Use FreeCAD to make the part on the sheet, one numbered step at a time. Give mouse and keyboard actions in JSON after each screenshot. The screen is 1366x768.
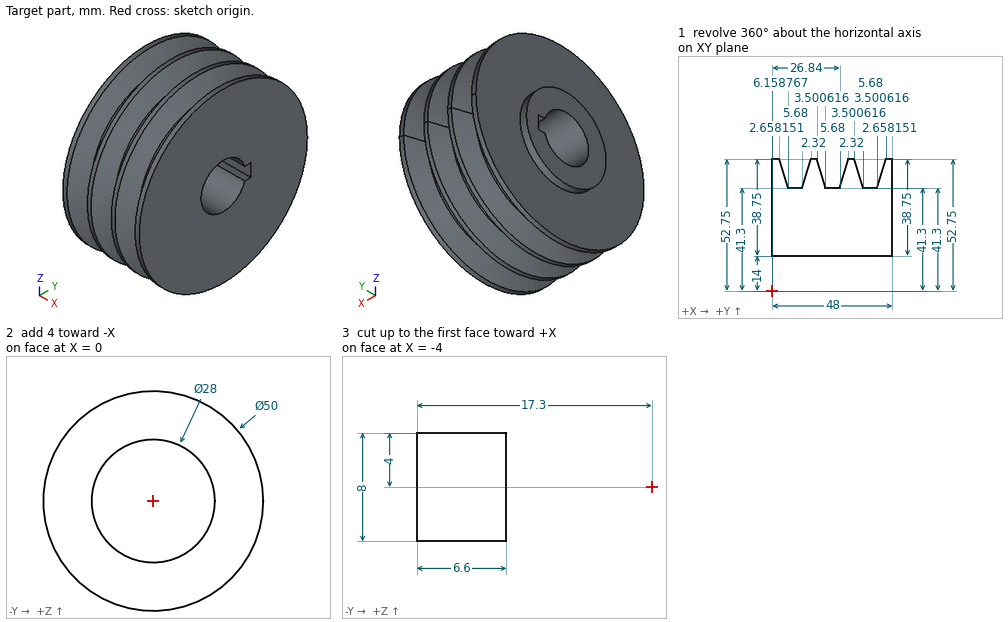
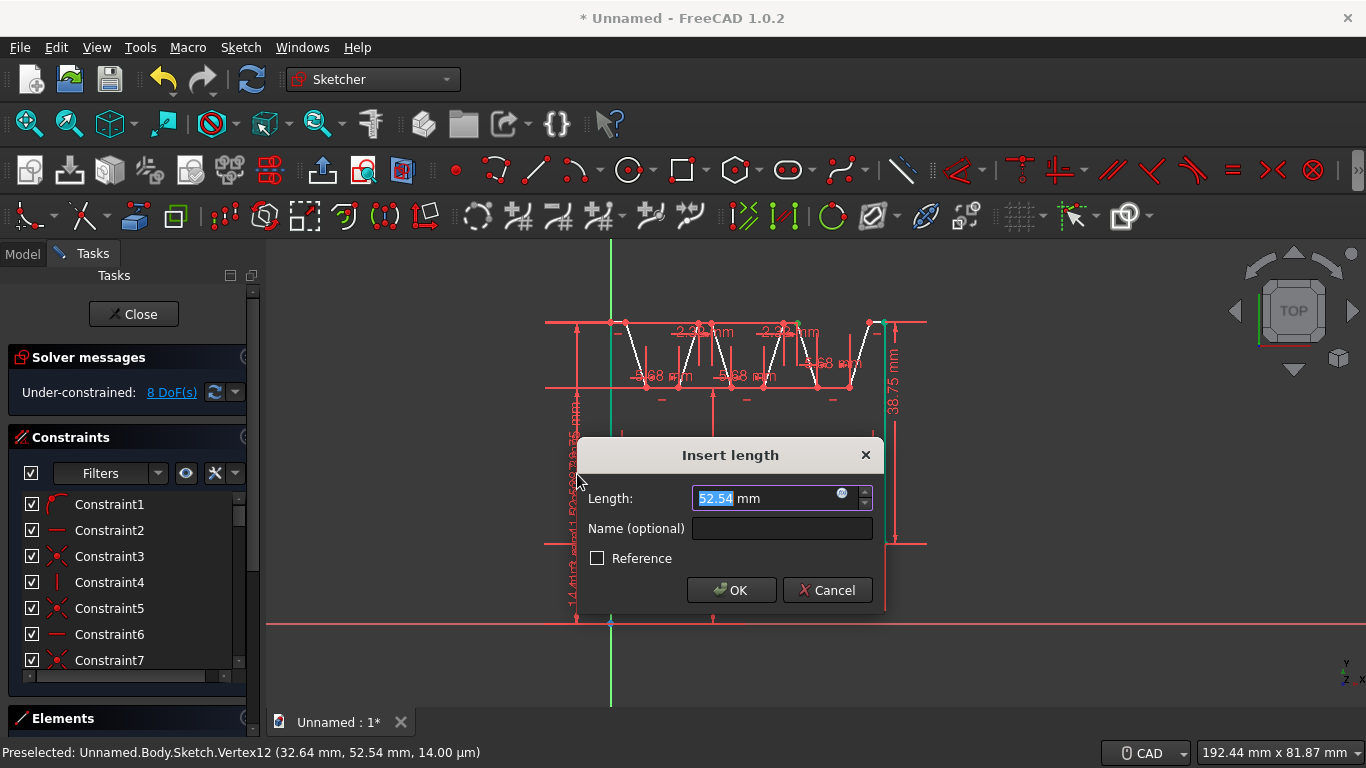
{"action": "type", "text": "52.75"}
{"action": "key", "text": "Return"}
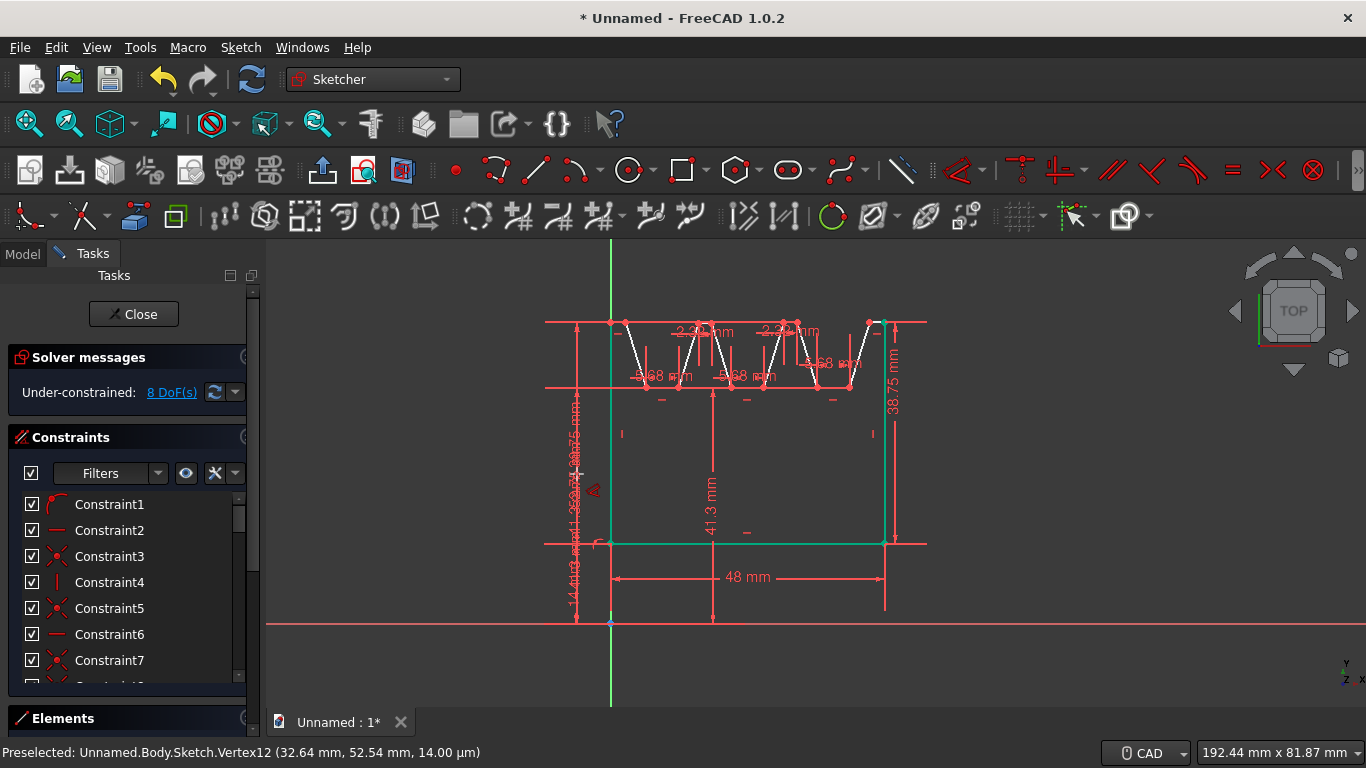
{"action": "left_click", "coordinate": [764, 388]}
{"action": "left_click", "coordinate": [687, 658]}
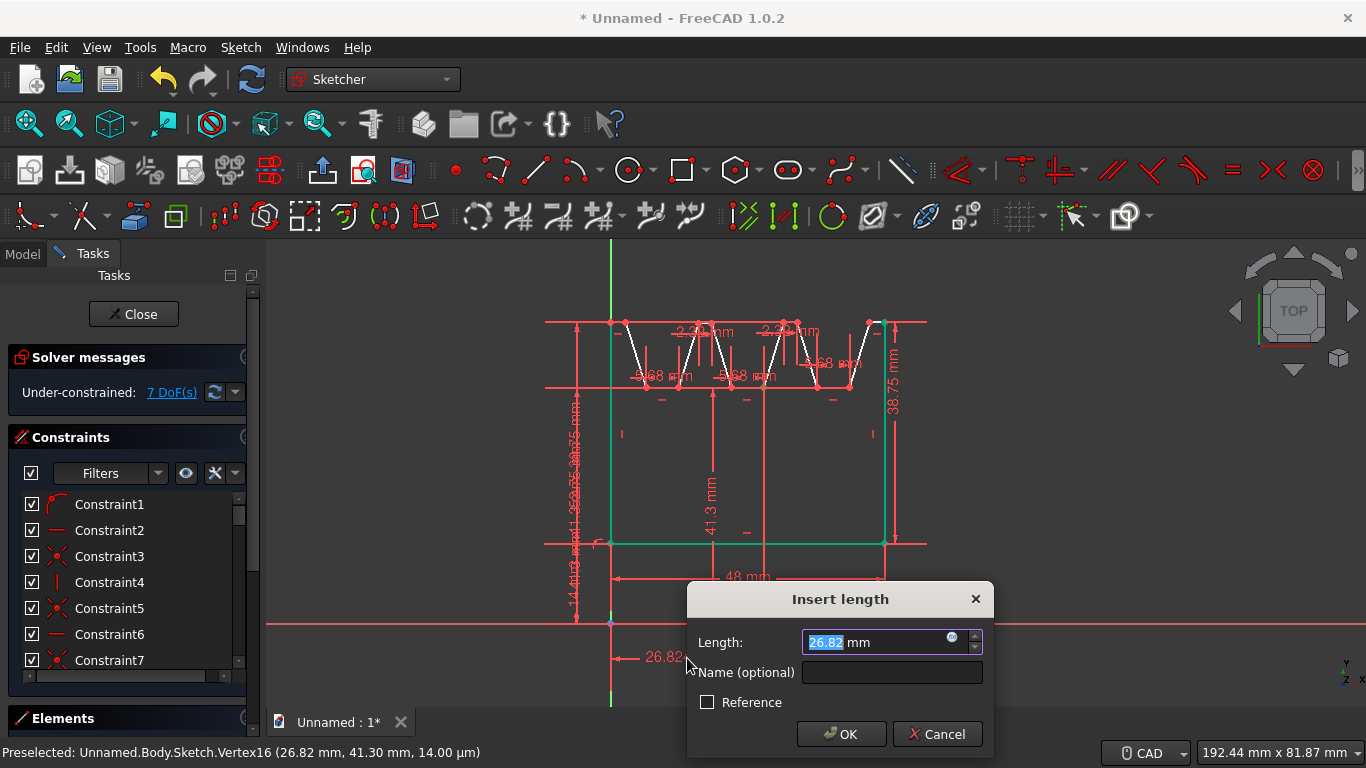
{"action": "type", "text": "26.84"}
{"action": "key", "text": "Return"}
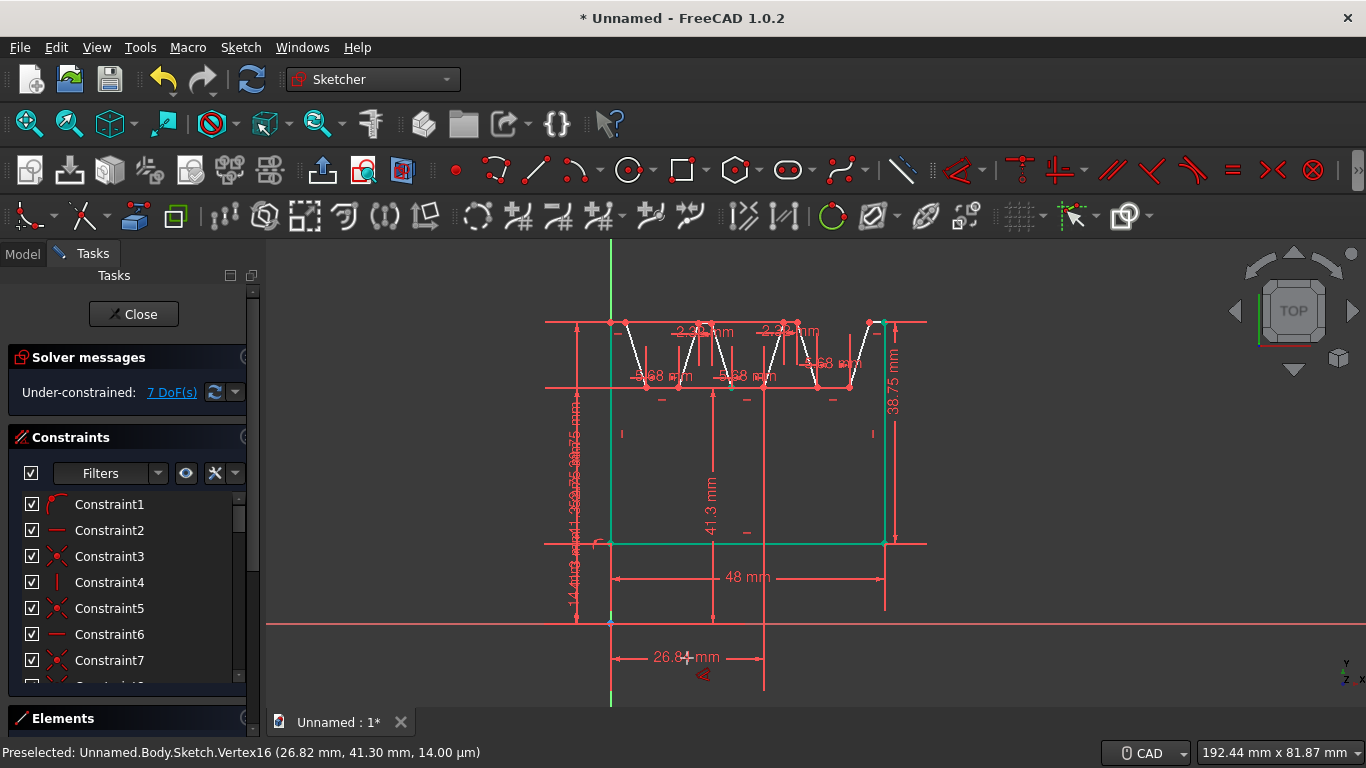
{"action": "left_click", "coordinate": [712, 323]}
{"action": "left_click", "coordinate": [577, 405]}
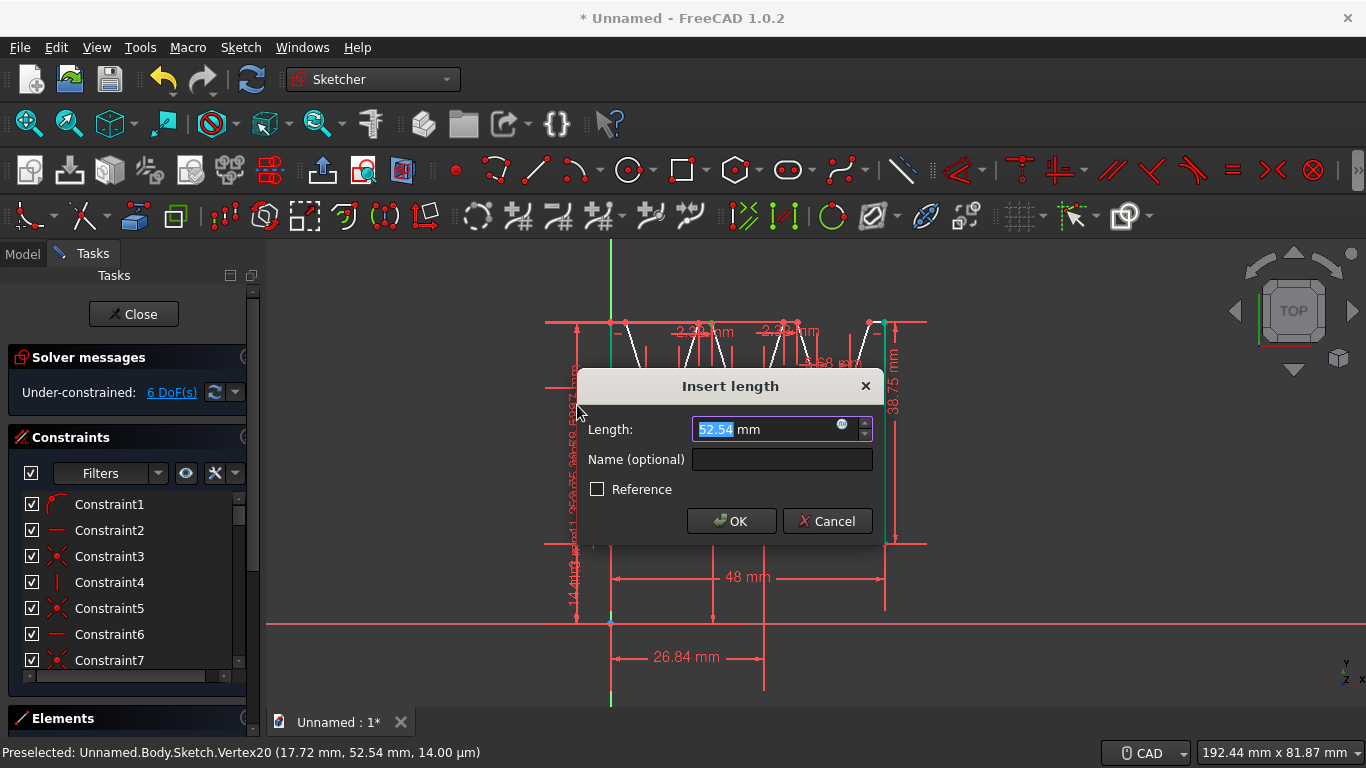
{"action": "type", "text": "52.75"}
{"action": "key", "text": "Return"}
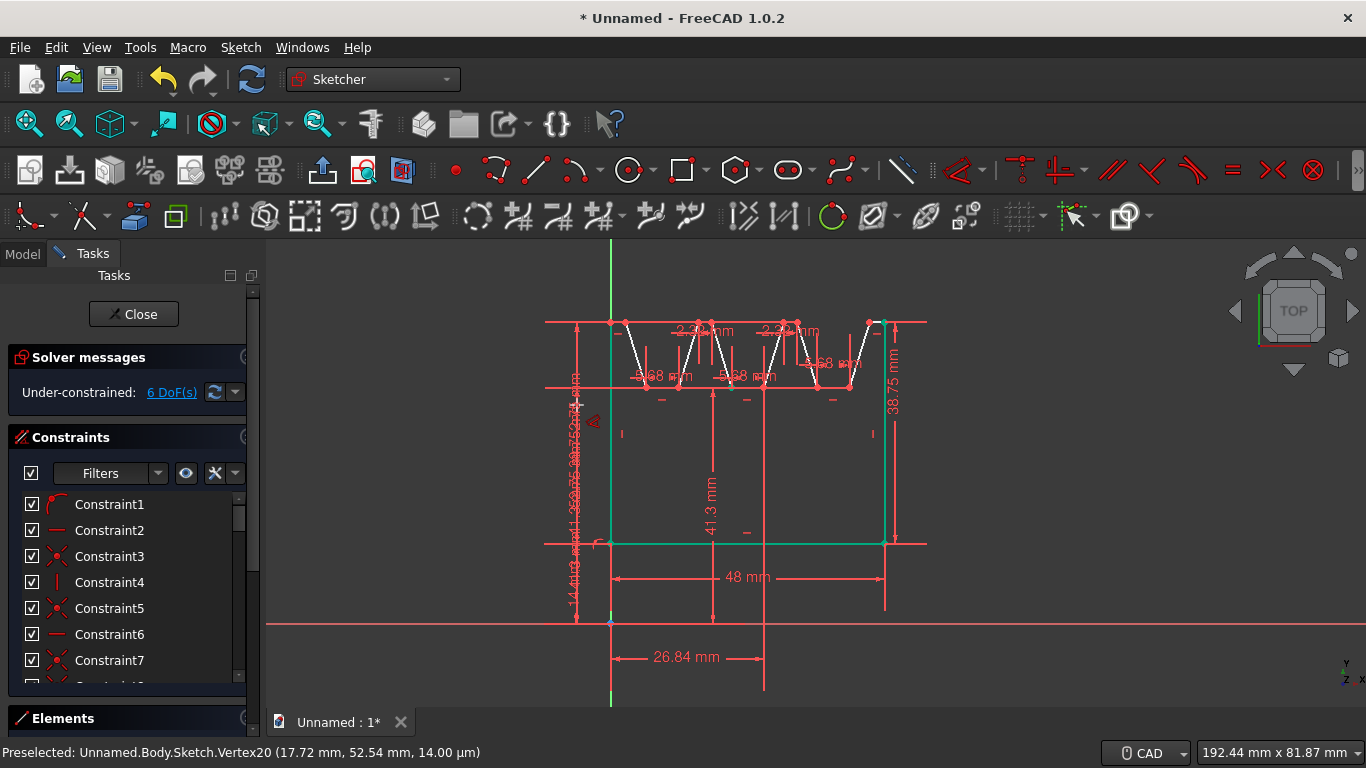
{"action": "scroll", "coordinate": [877, 322], "scroll_direction": "up", "scroll_amount": 5}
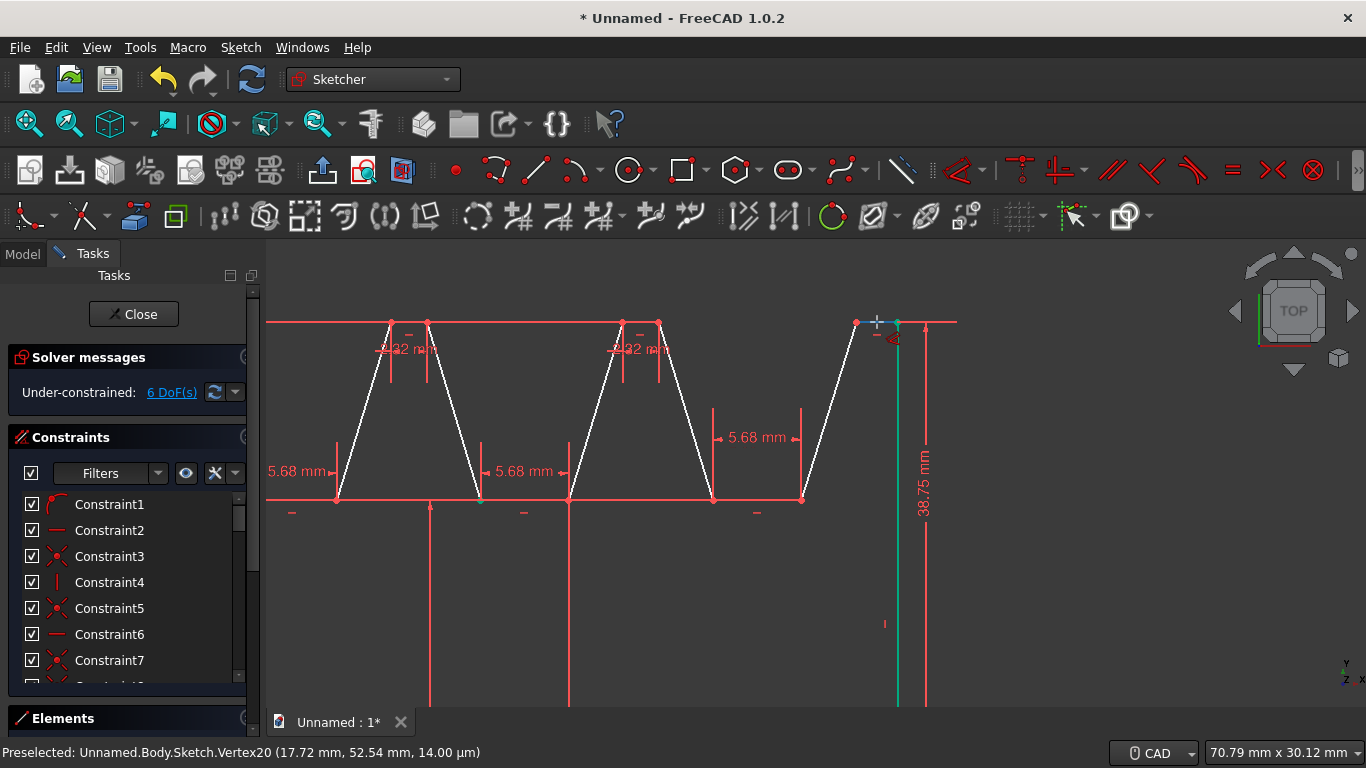
{"action": "left_click", "coordinate": [877, 322]}
{"action": "left_click", "coordinate": [877, 288]}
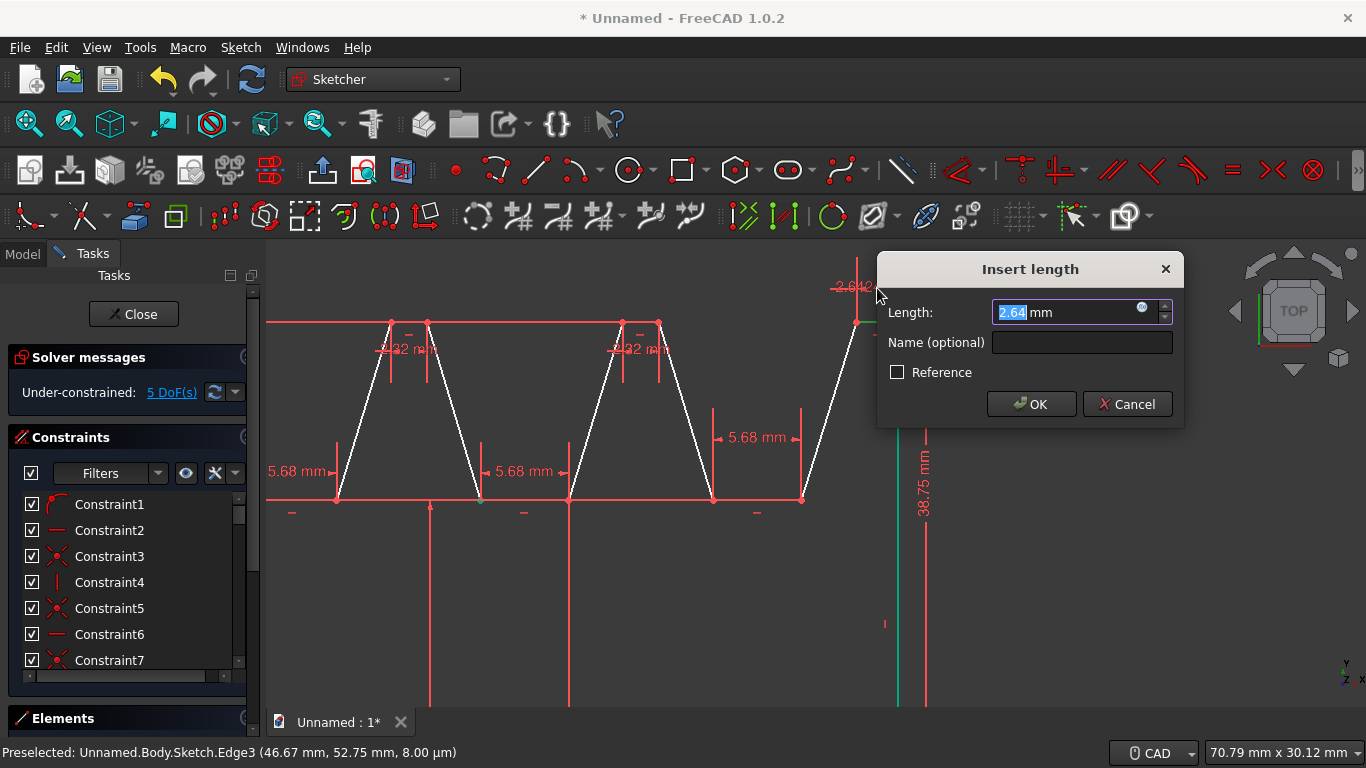
{"action": "type", "text": "2.658151"}
{"action": "key", "text": "Return"}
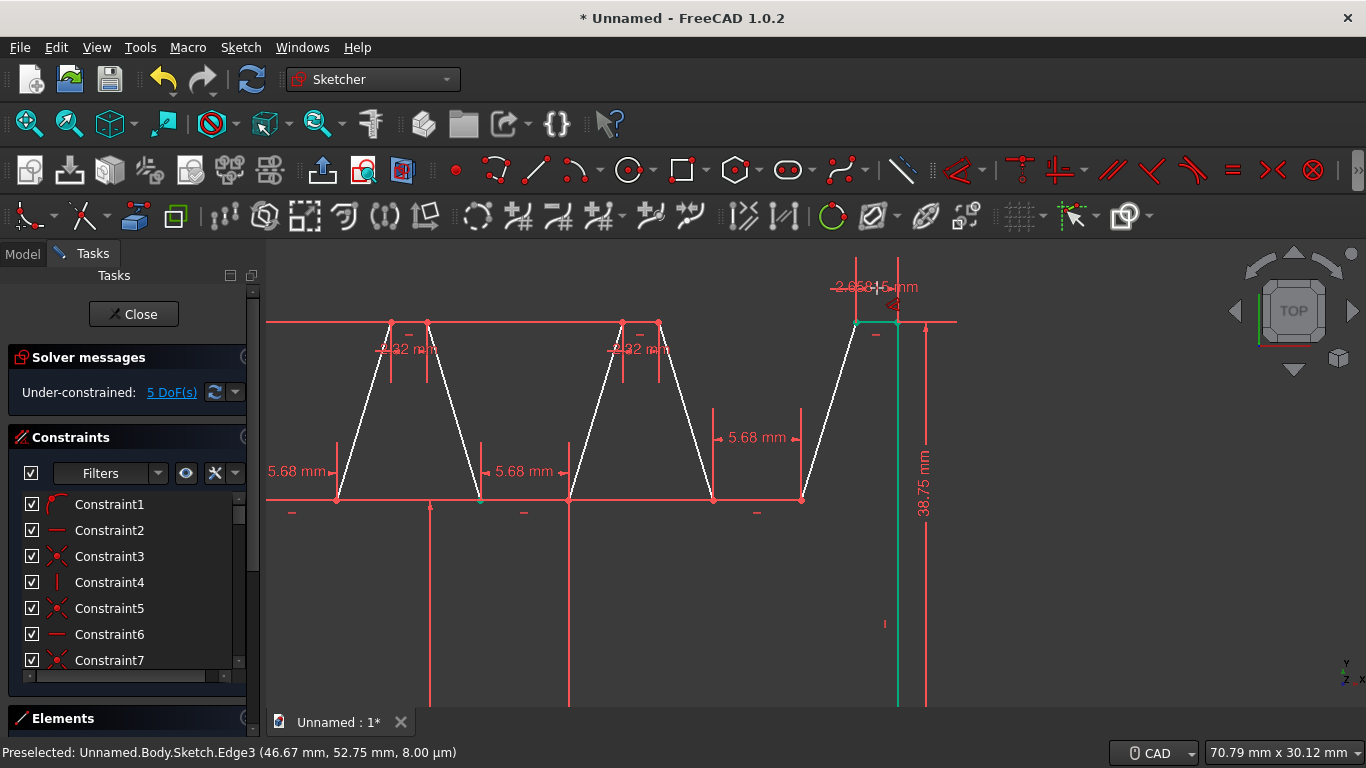
{"action": "scroll", "coordinate": [877, 322], "scroll_direction": "down", "scroll_amount": 5}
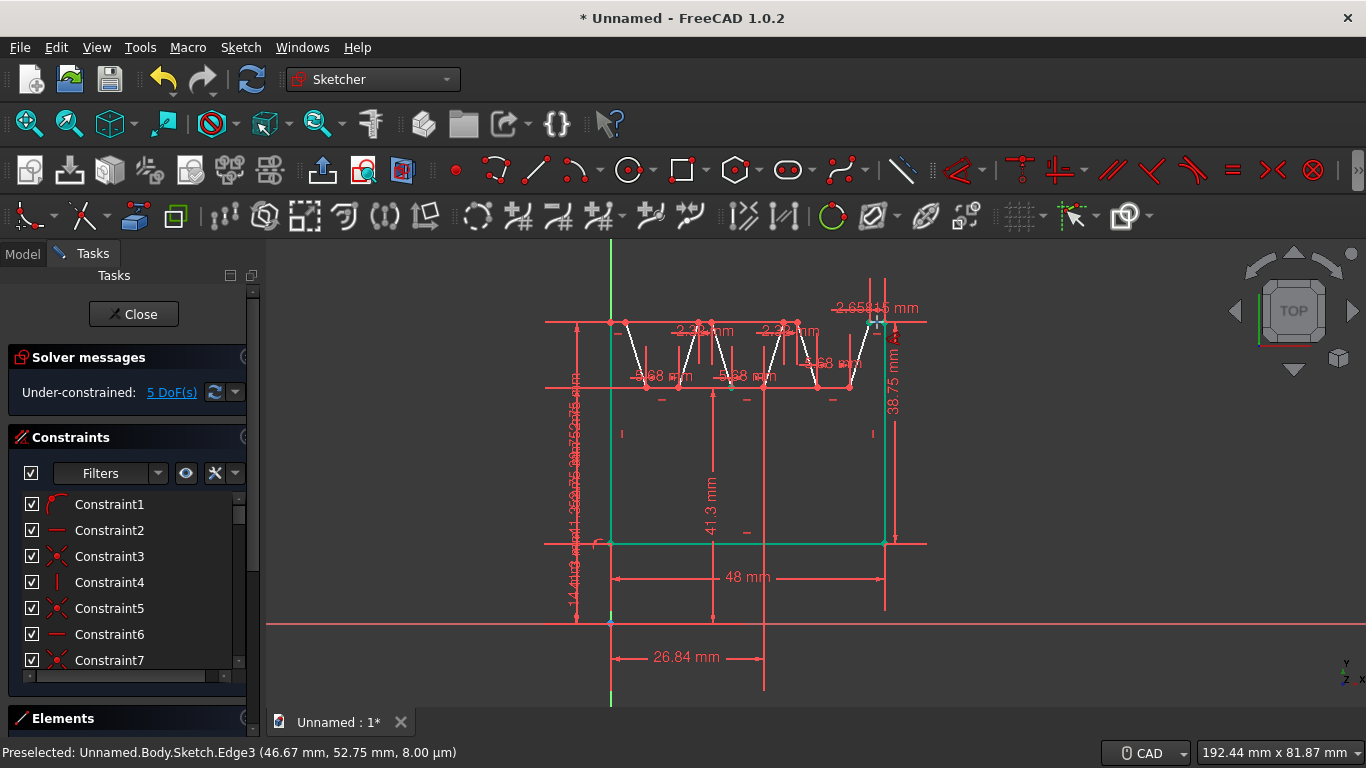
{"action": "scroll", "coordinate": [621, 322], "scroll_direction": "up", "scroll_amount": 6}